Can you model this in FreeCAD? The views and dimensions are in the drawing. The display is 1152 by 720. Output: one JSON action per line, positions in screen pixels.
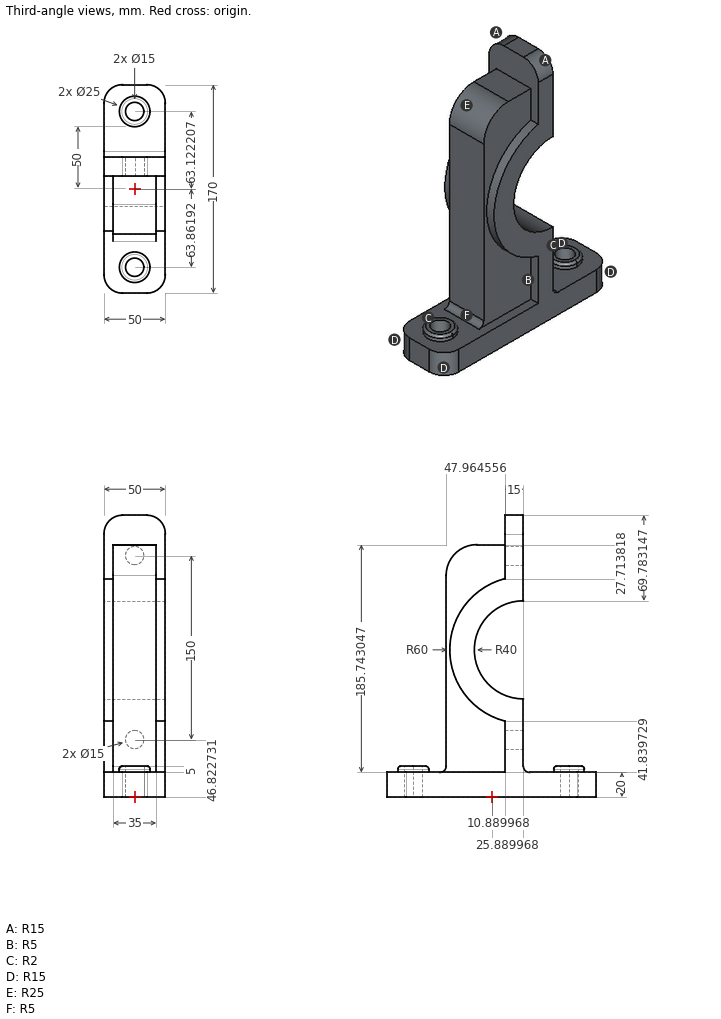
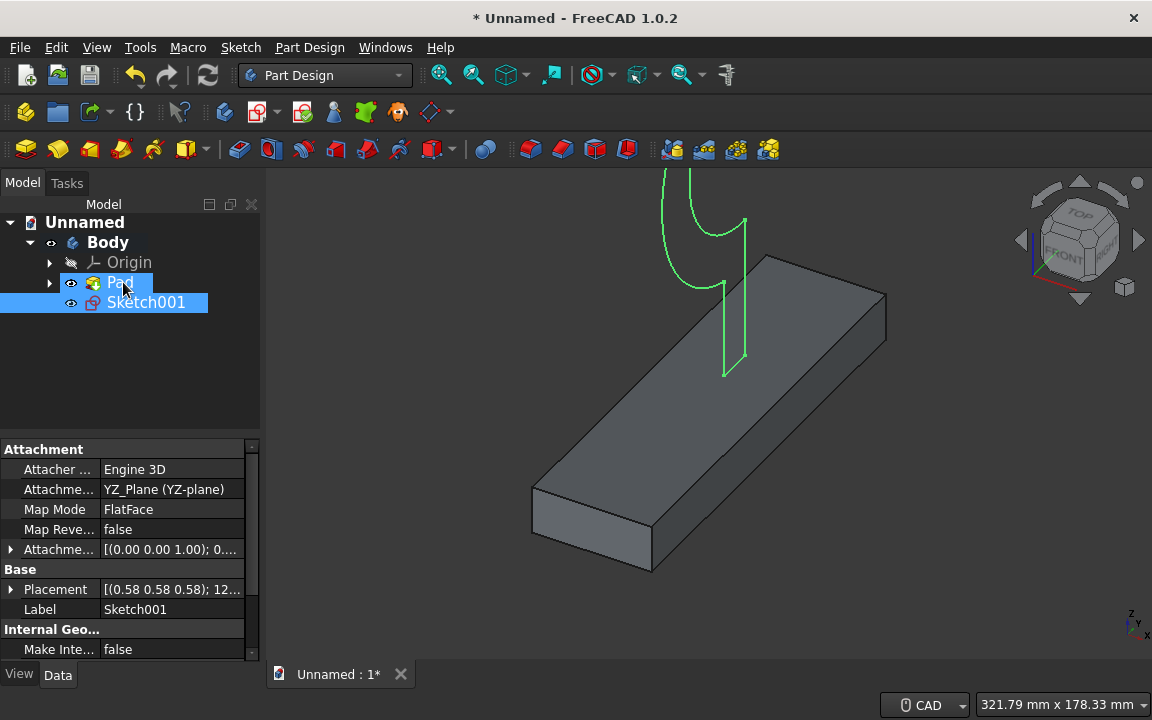
{"action": "left_click", "coordinate": [26, 150]}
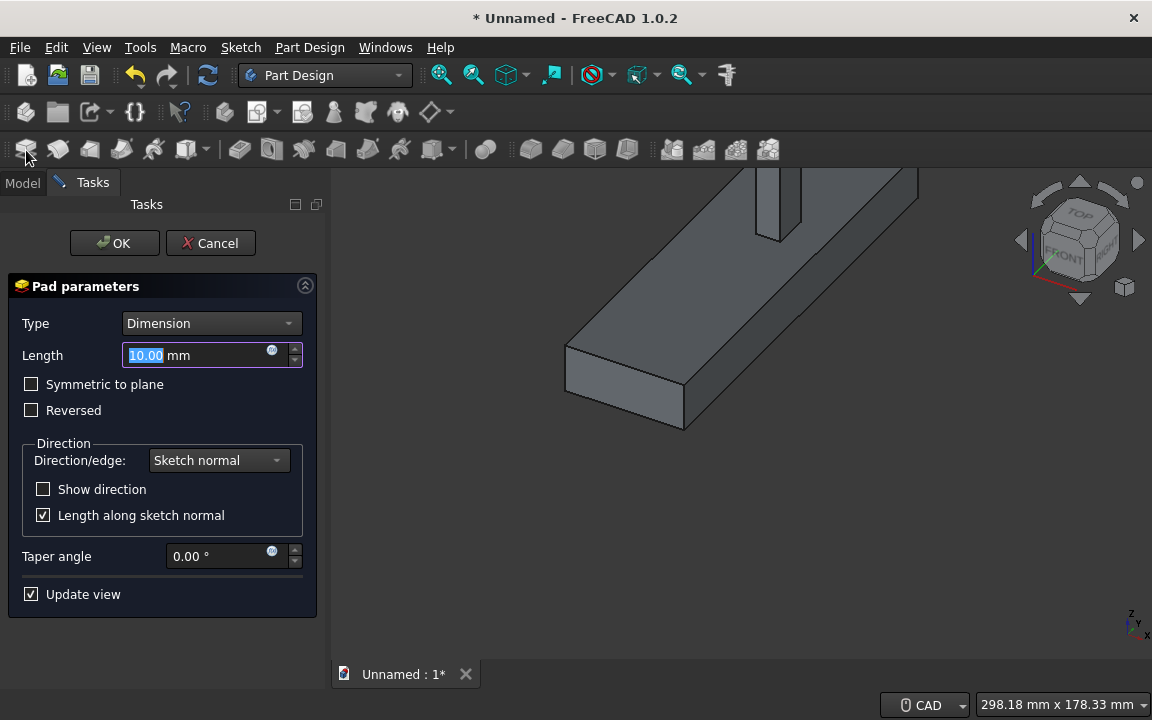
{"action": "type", "text": "50"}
{"action": "key", "text": "Tab"}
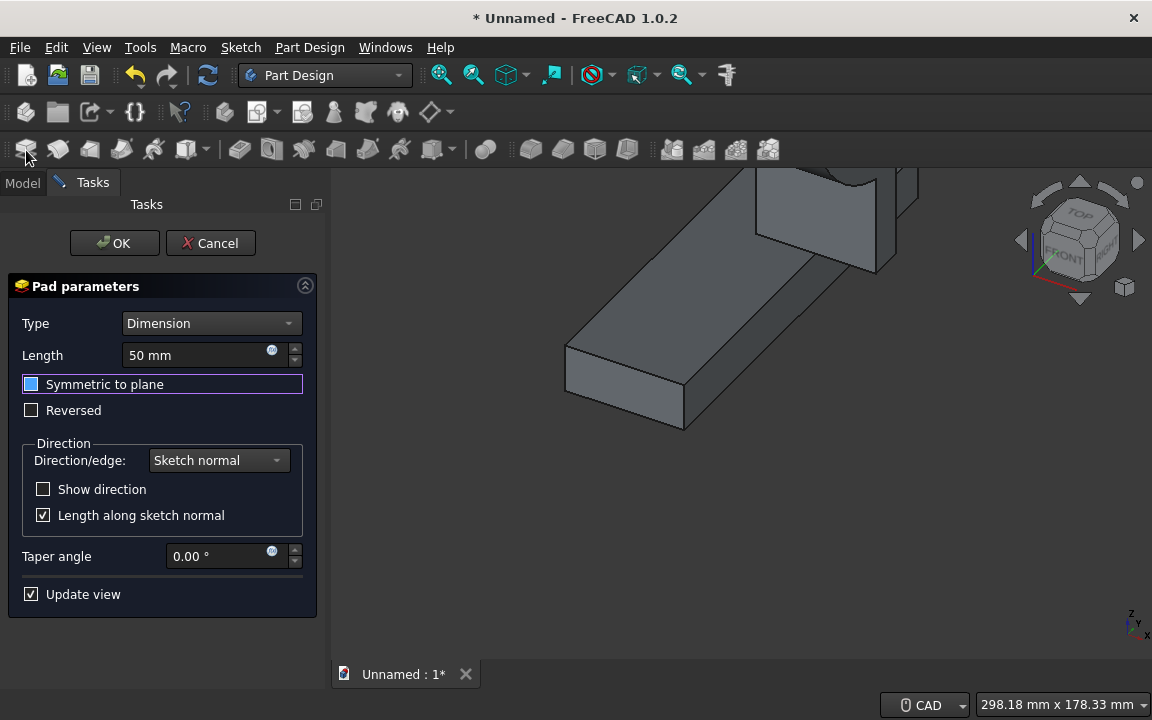
{"action": "left_click", "coordinate": [30, 384]}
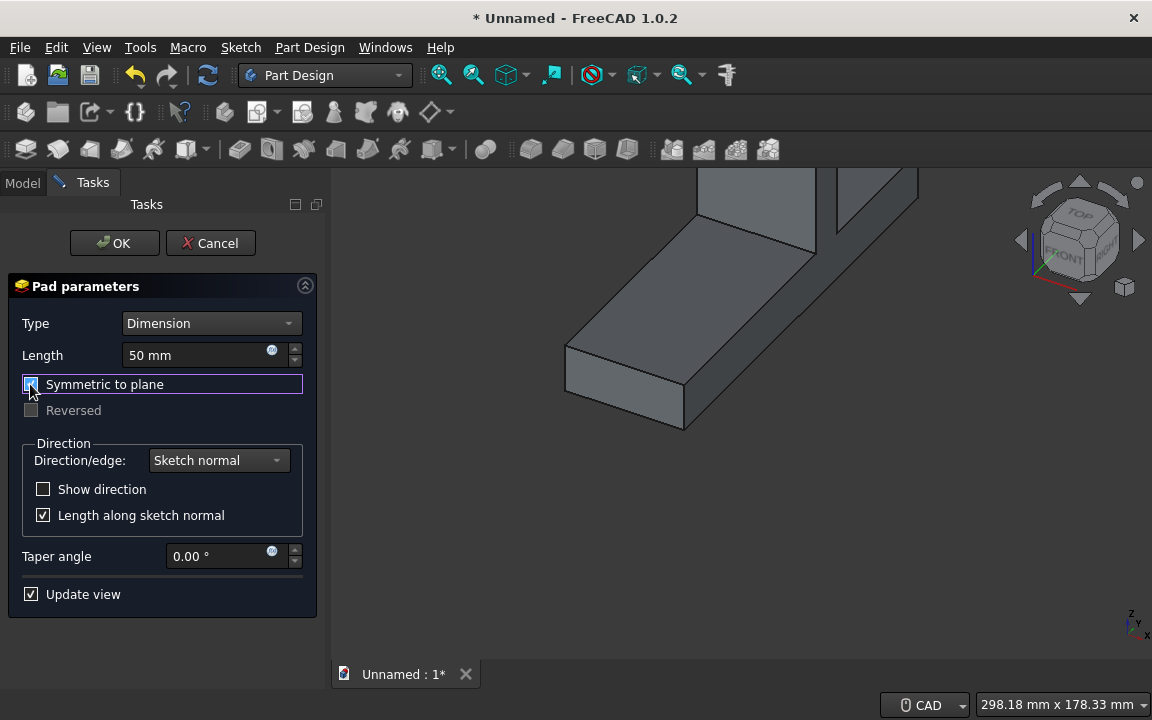
{"action": "left_click", "coordinate": [115, 243]}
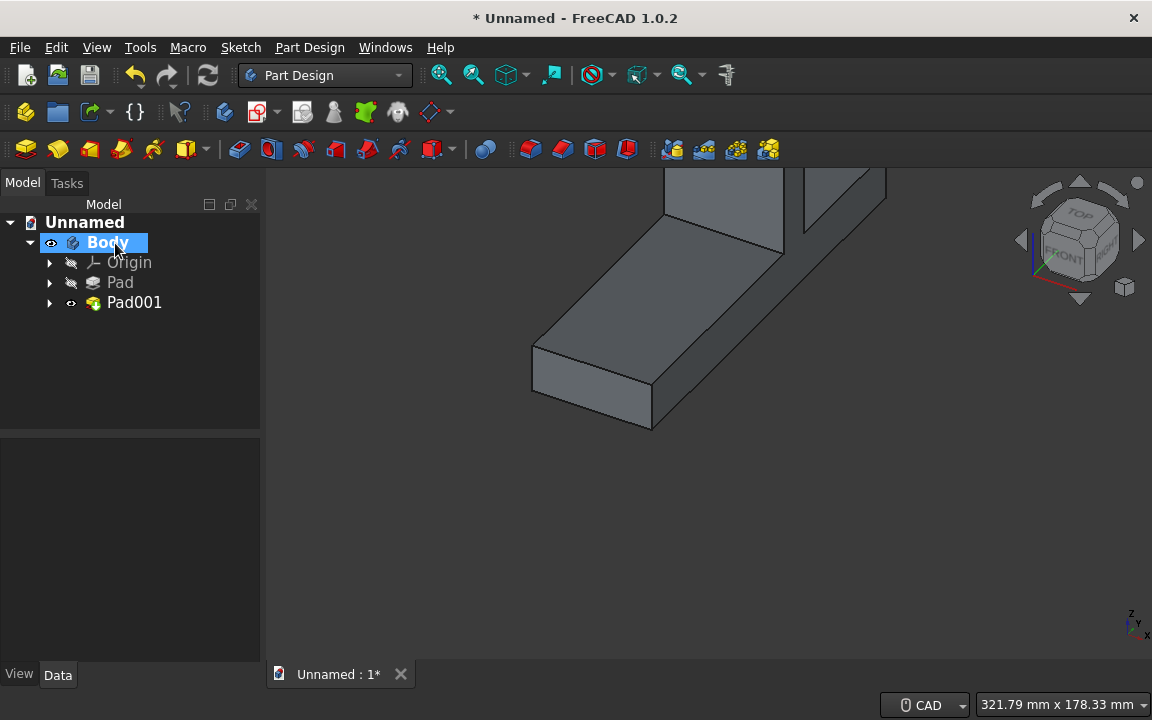
{"action": "key", "text": "v f"}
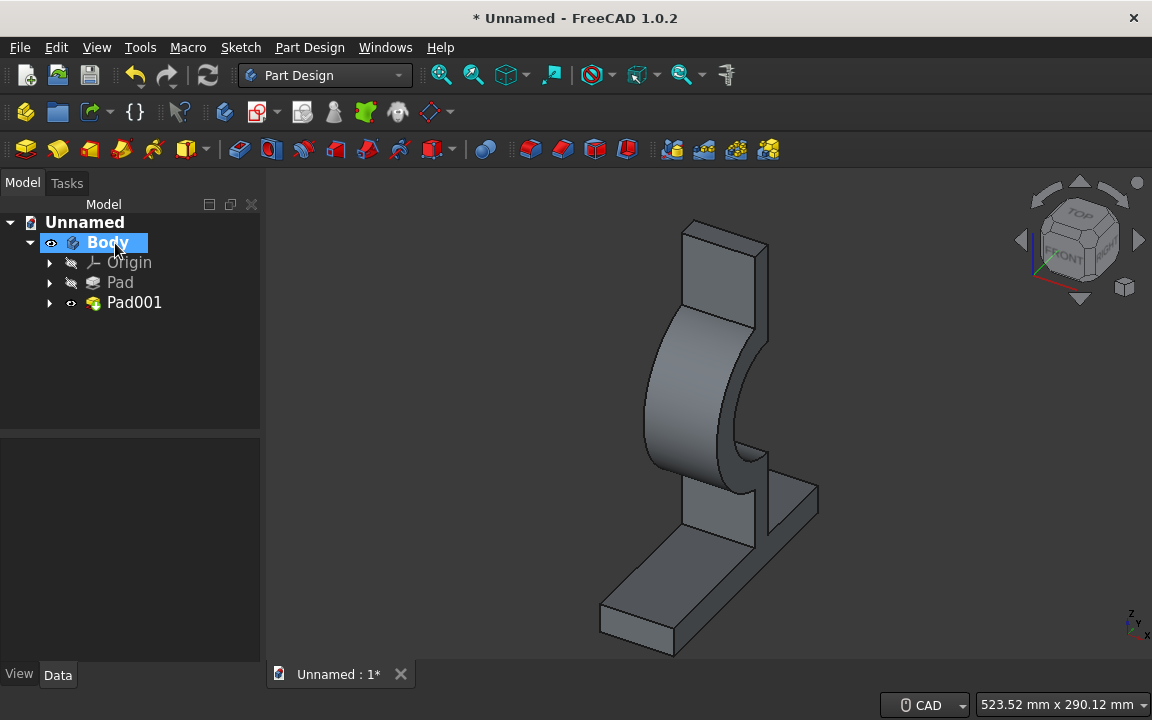
{"action": "left_click", "coordinate": [761, 250]}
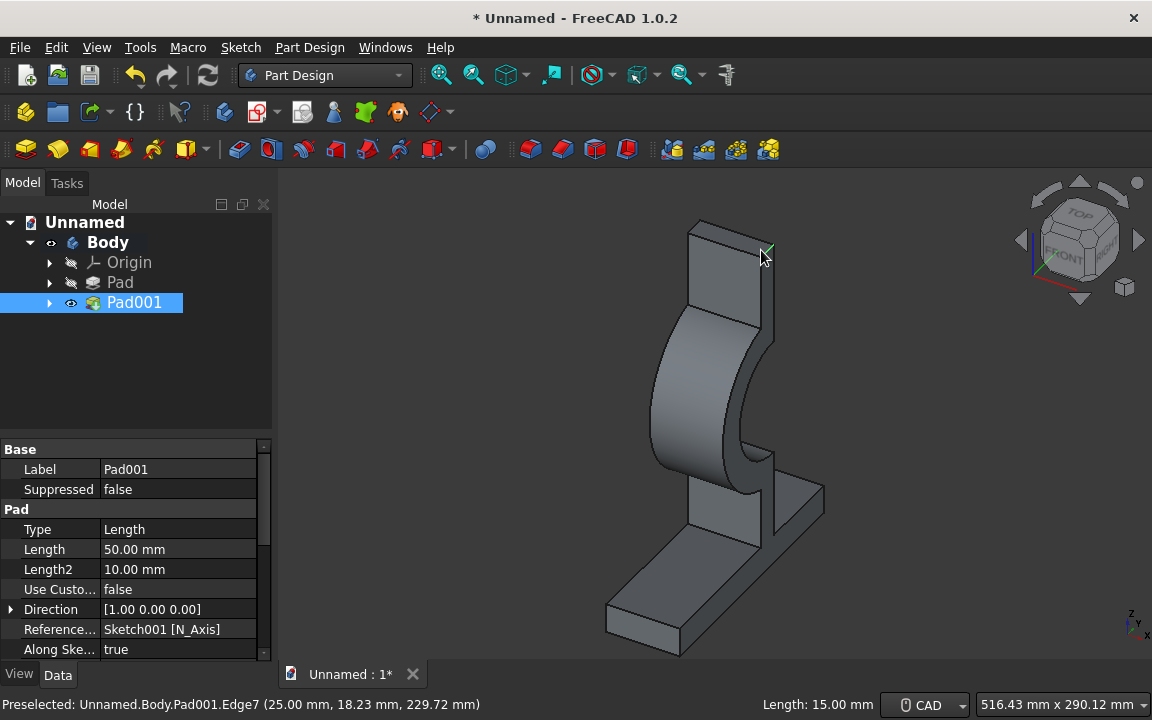
{"action": "key", "text": "0"}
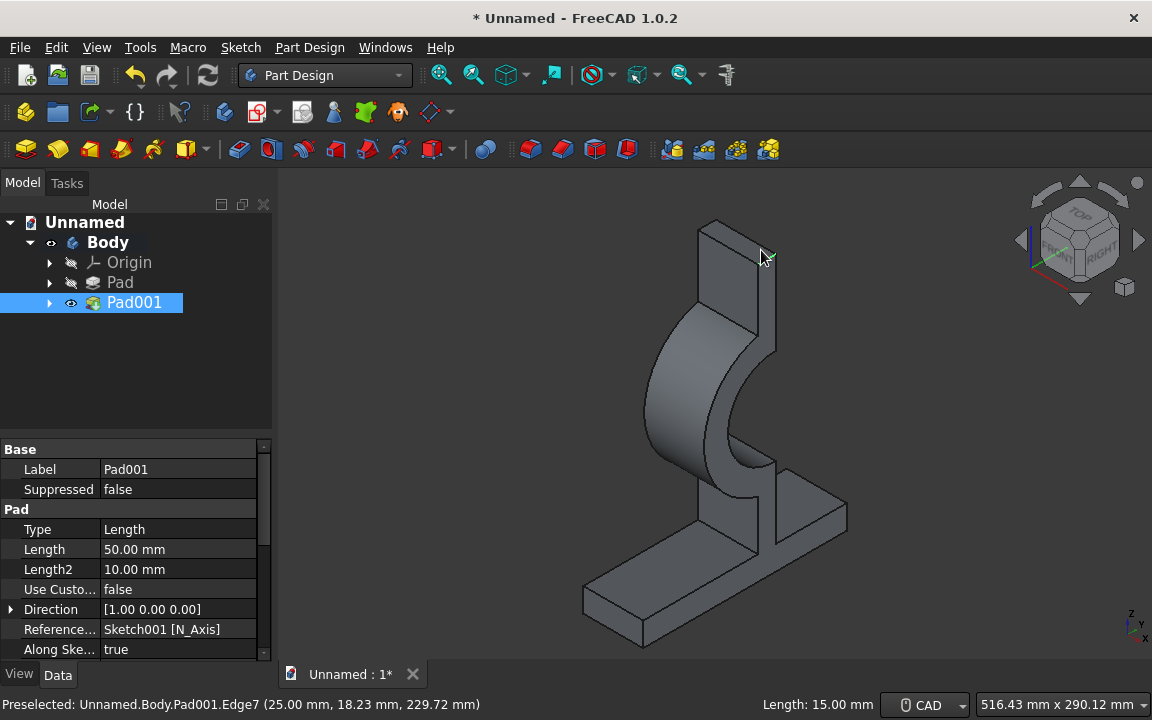
{"action": "key", "text": "2"}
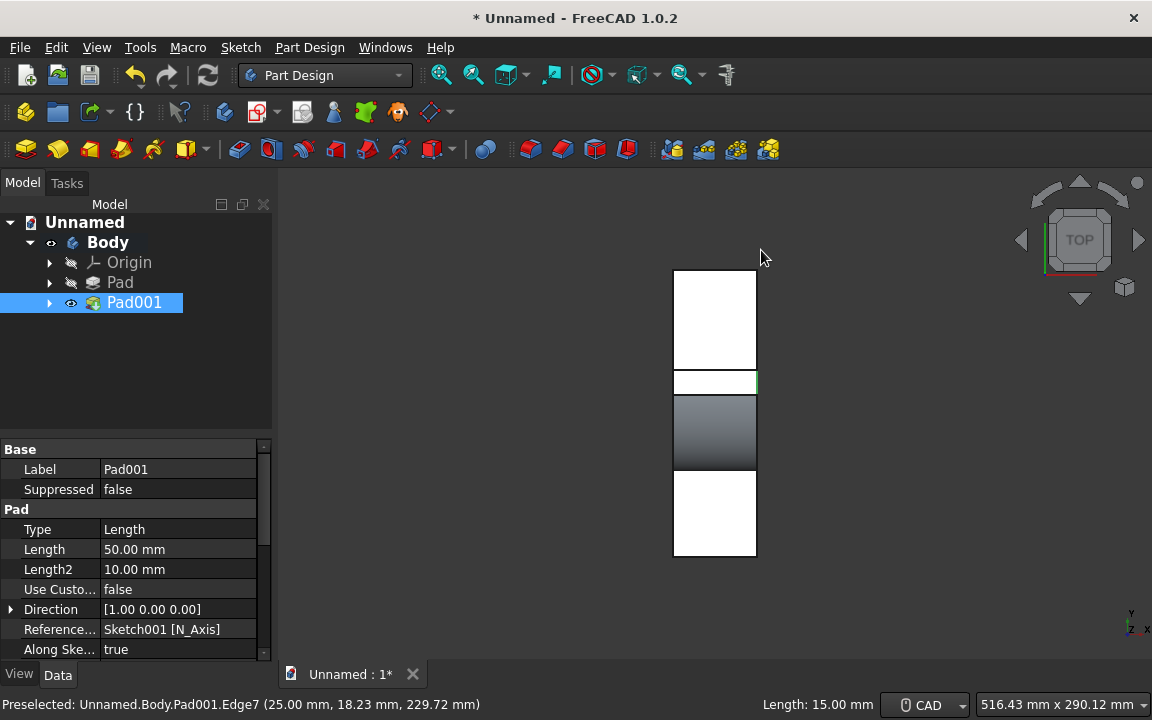
{"action": "left_click", "coordinate": [673, 381], "text": "ctrl"}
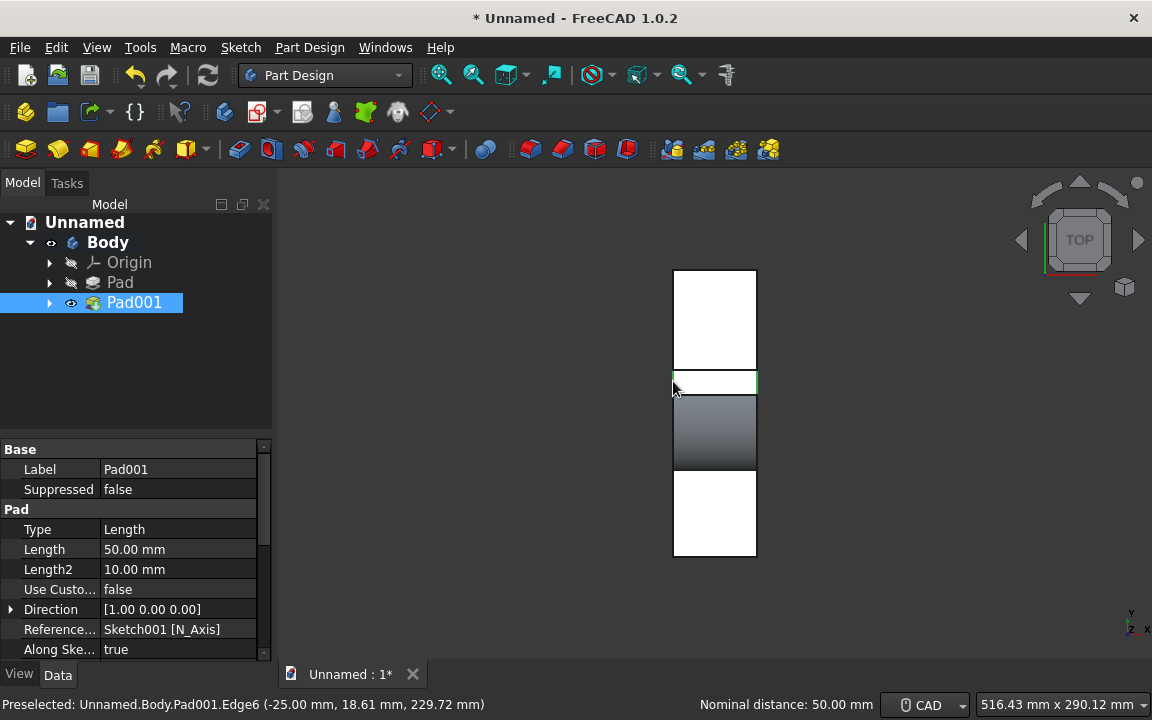
{"action": "left_click", "coordinate": [532, 150]}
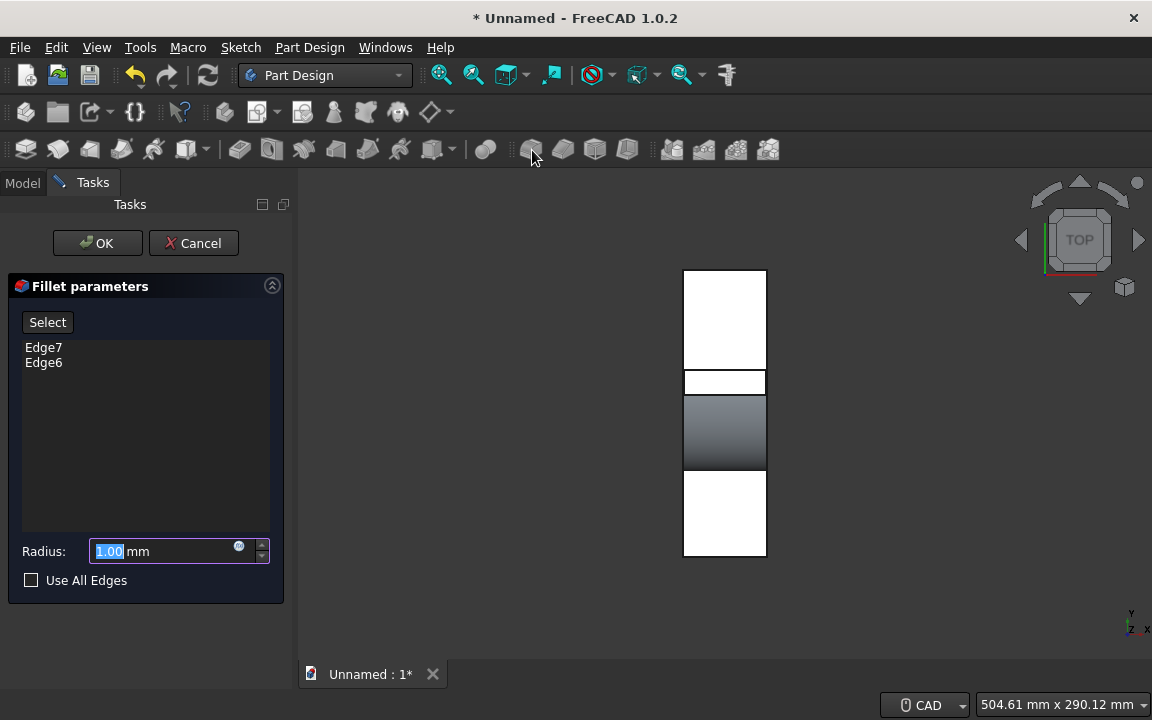
{"action": "type", "text": "15"}
{"action": "key", "text": "Tab"}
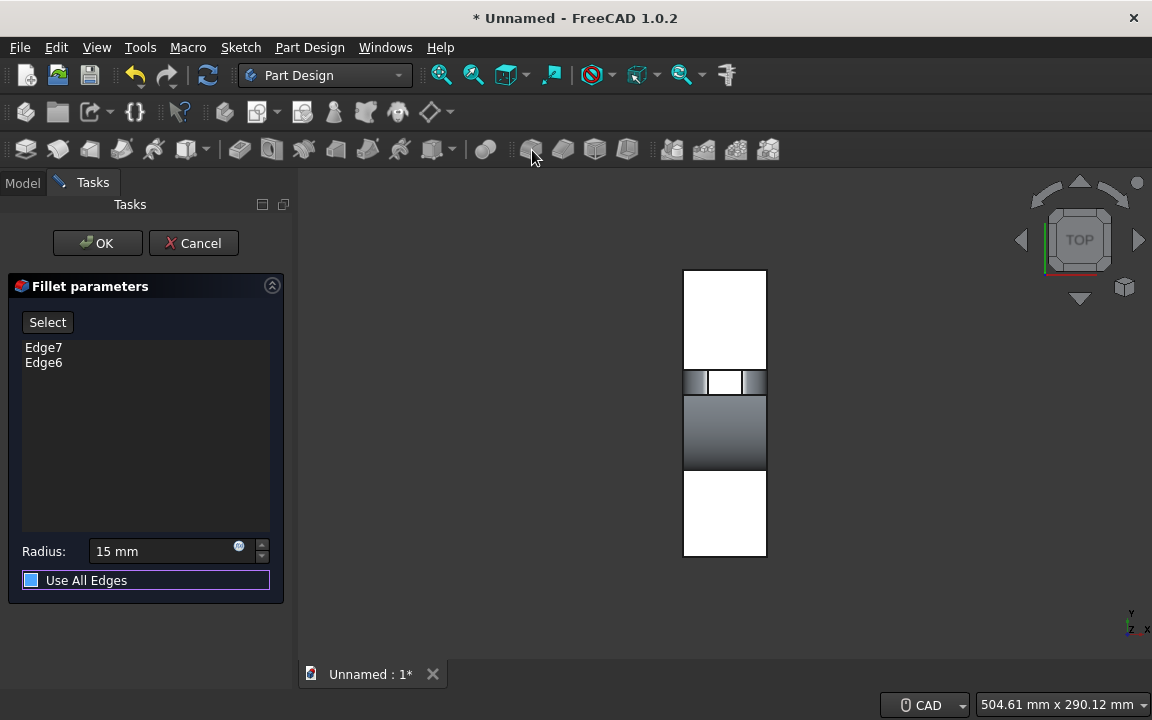
{"action": "left_click", "coordinate": [98, 243]}